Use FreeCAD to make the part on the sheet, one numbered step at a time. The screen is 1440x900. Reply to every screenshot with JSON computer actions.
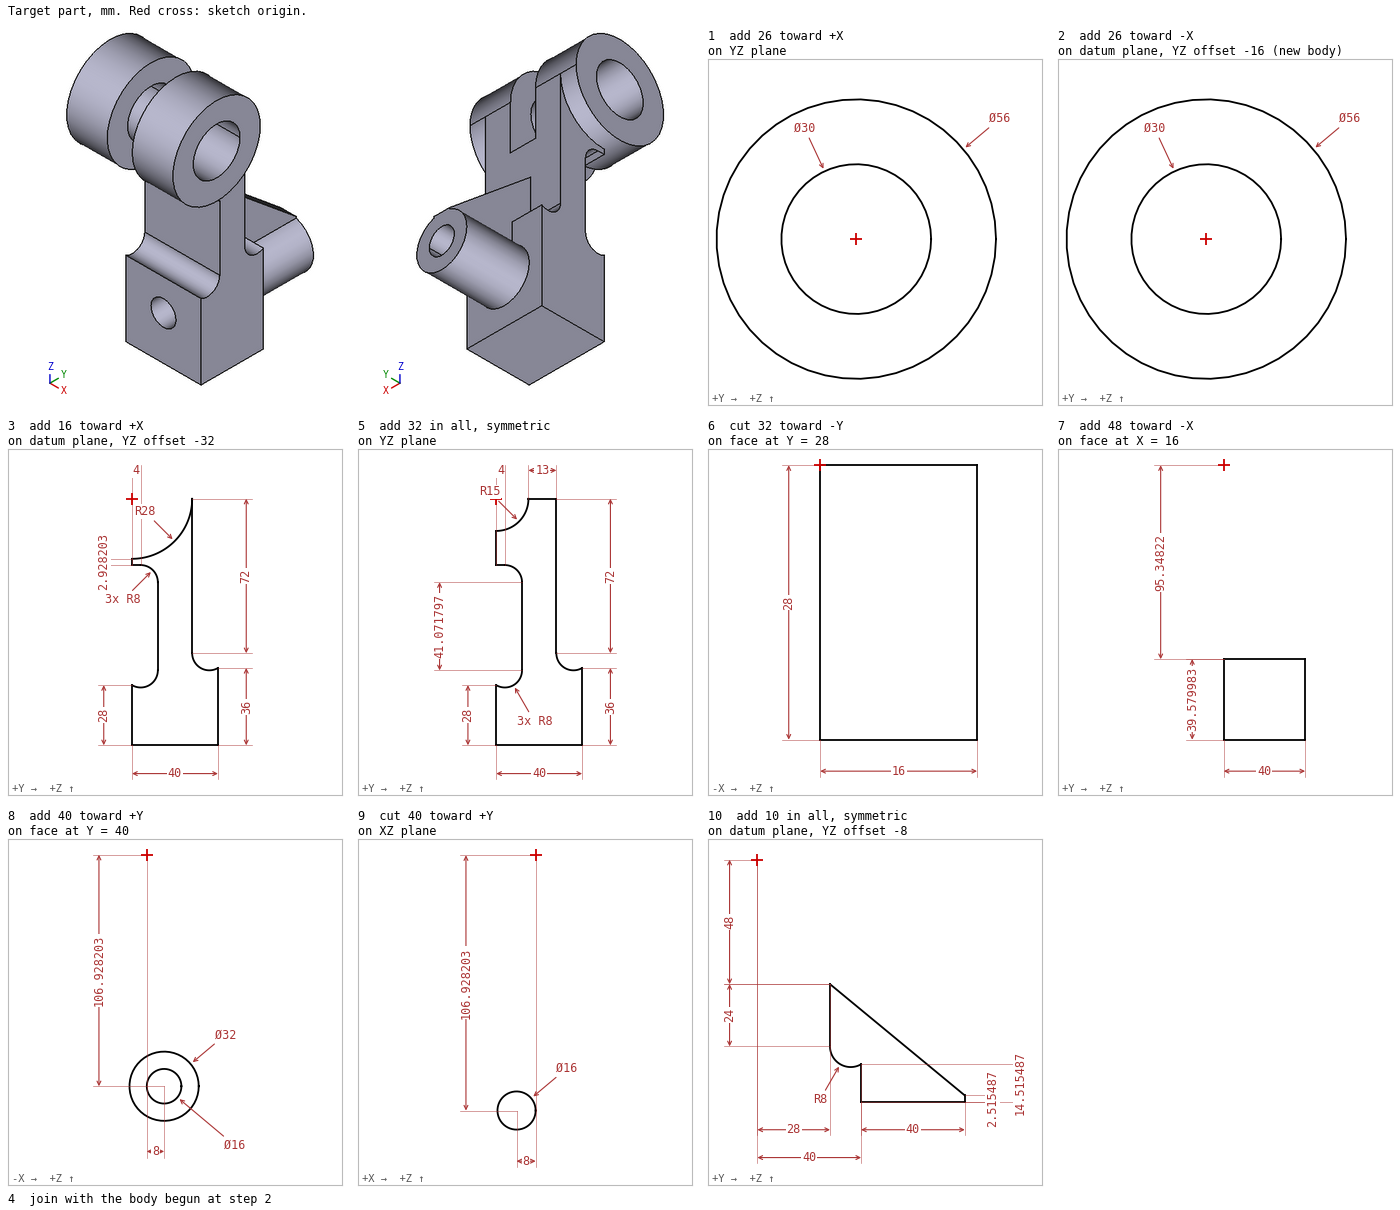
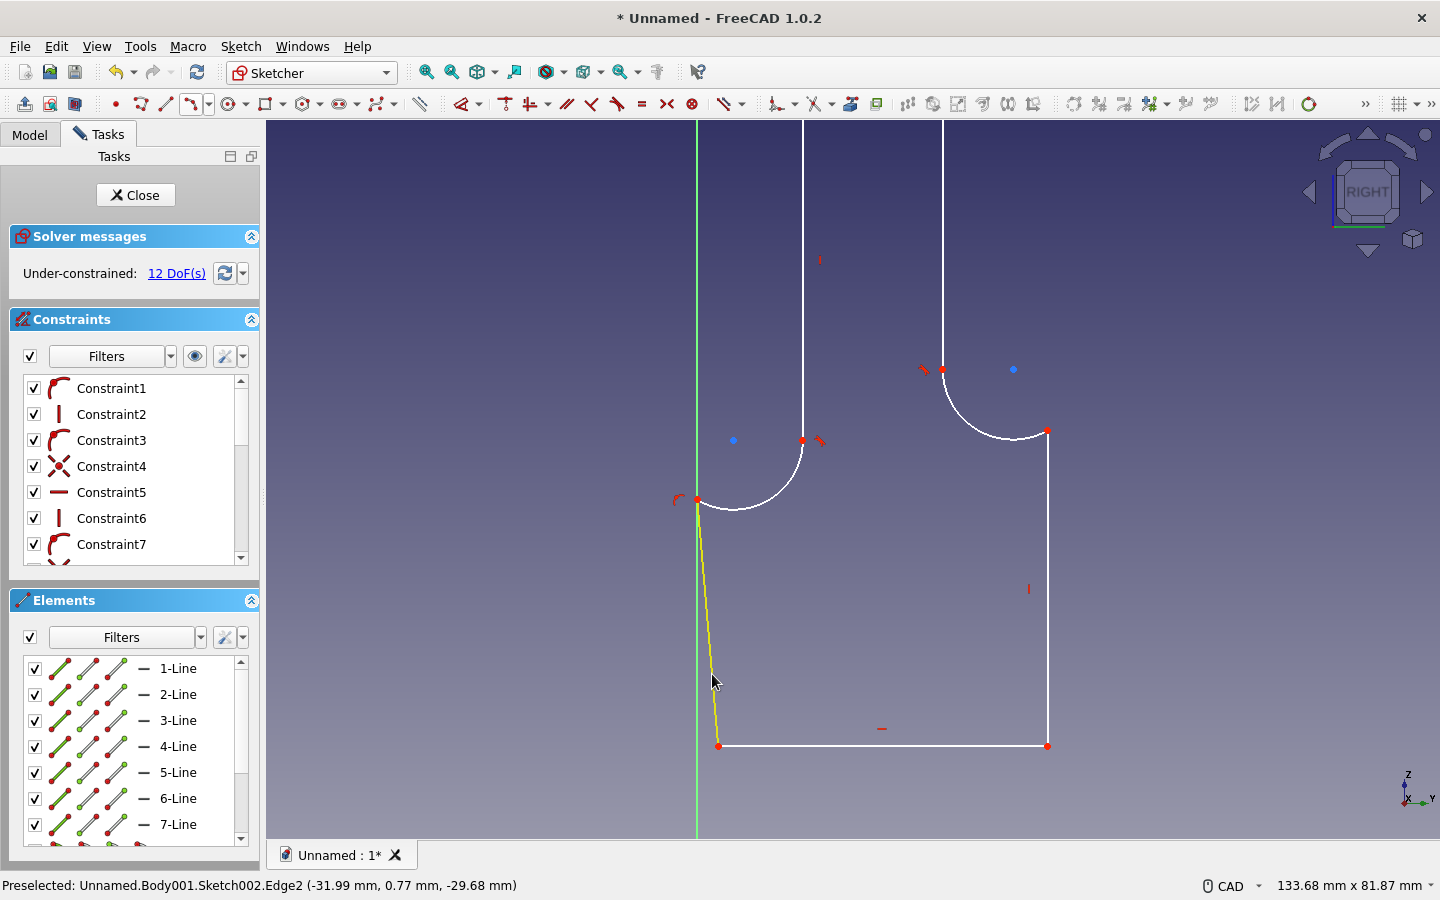
{"action": "left_click", "coordinate": [712, 672]}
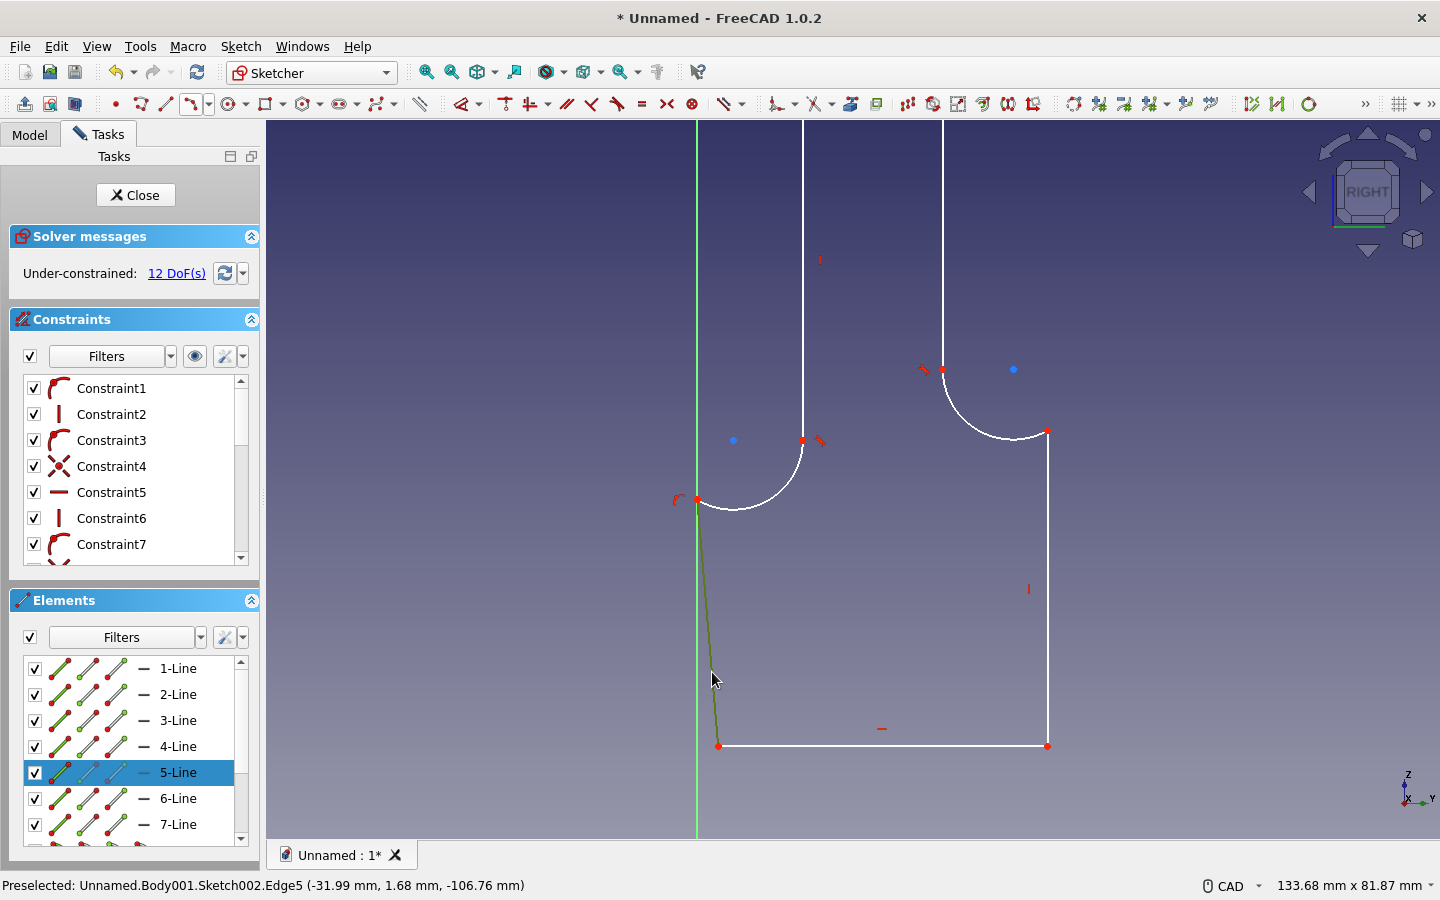
{"action": "left_click", "coordinate": [548, 104]}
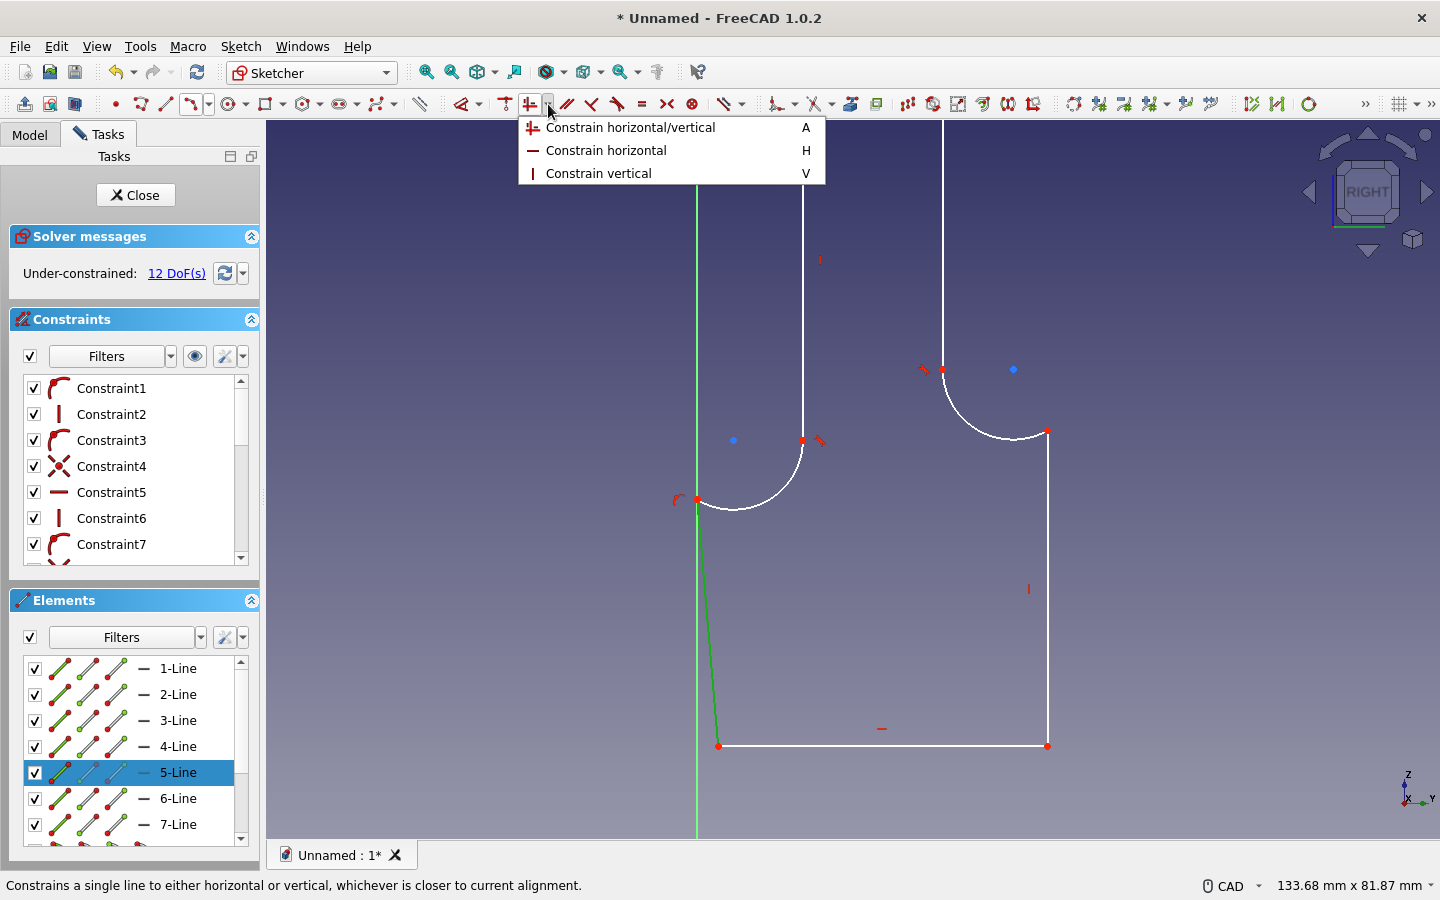
{"action": "left_click", "coordinate": [672, 174]}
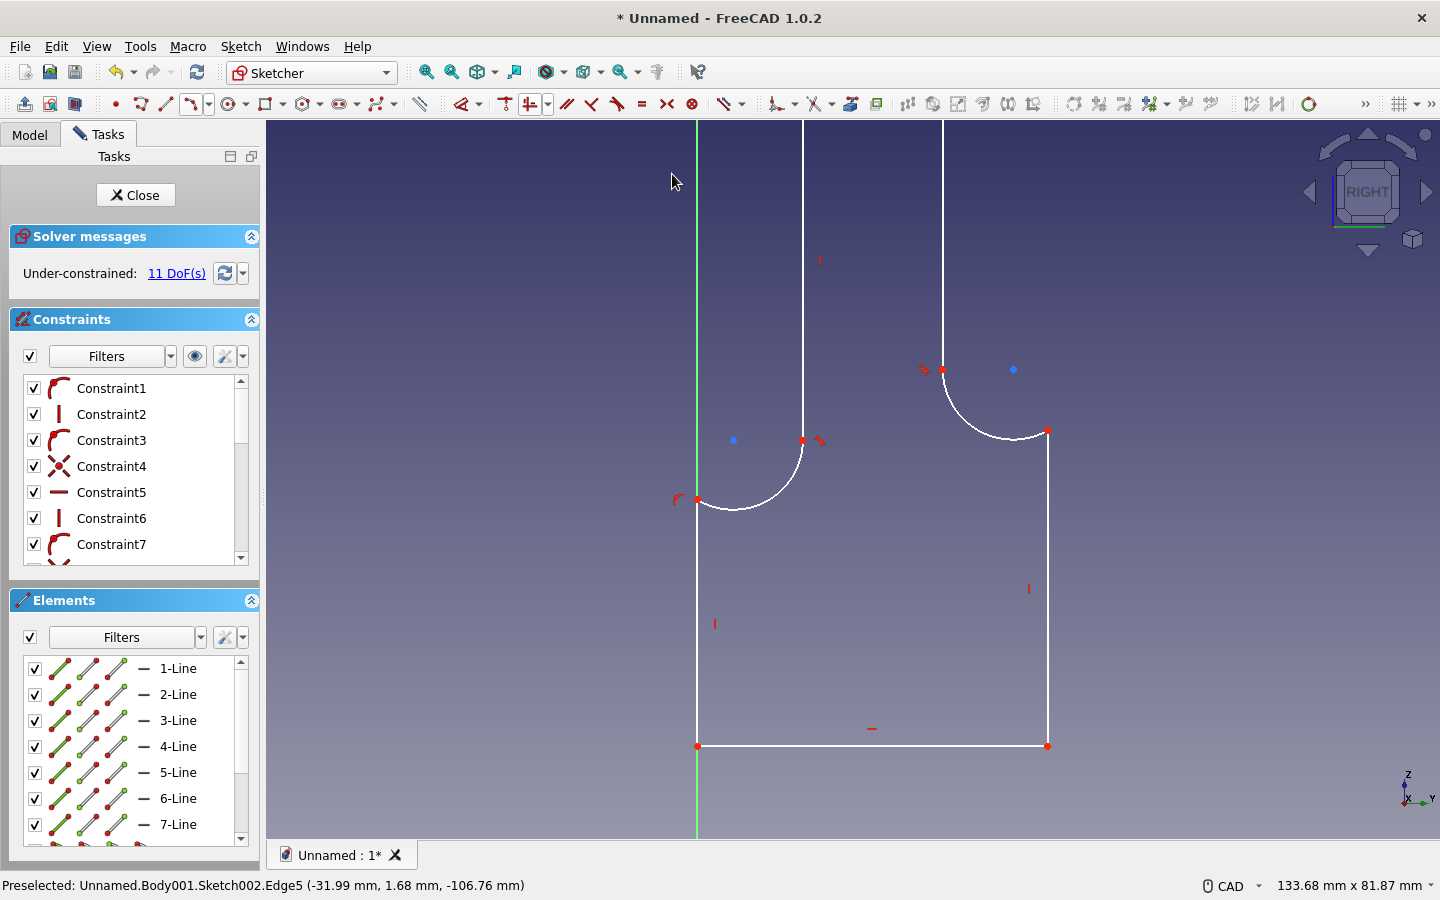
{"action": "scroll", "coordinate": [712, 675], "scroll_direction": "down", "scroll_amount": 4}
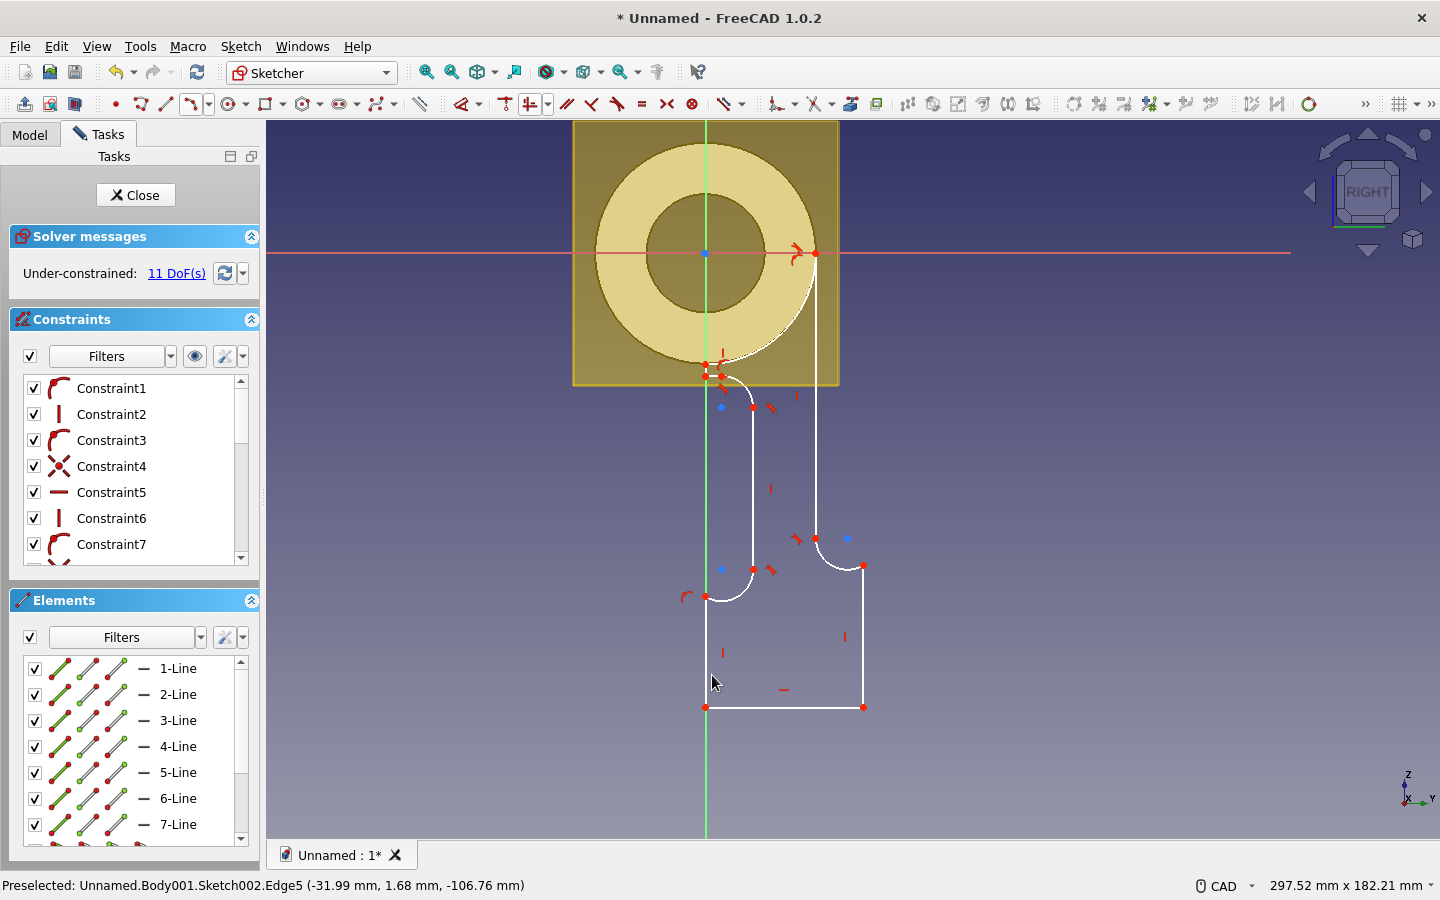
{"action": "left_click", "coordinate": [750, 393]}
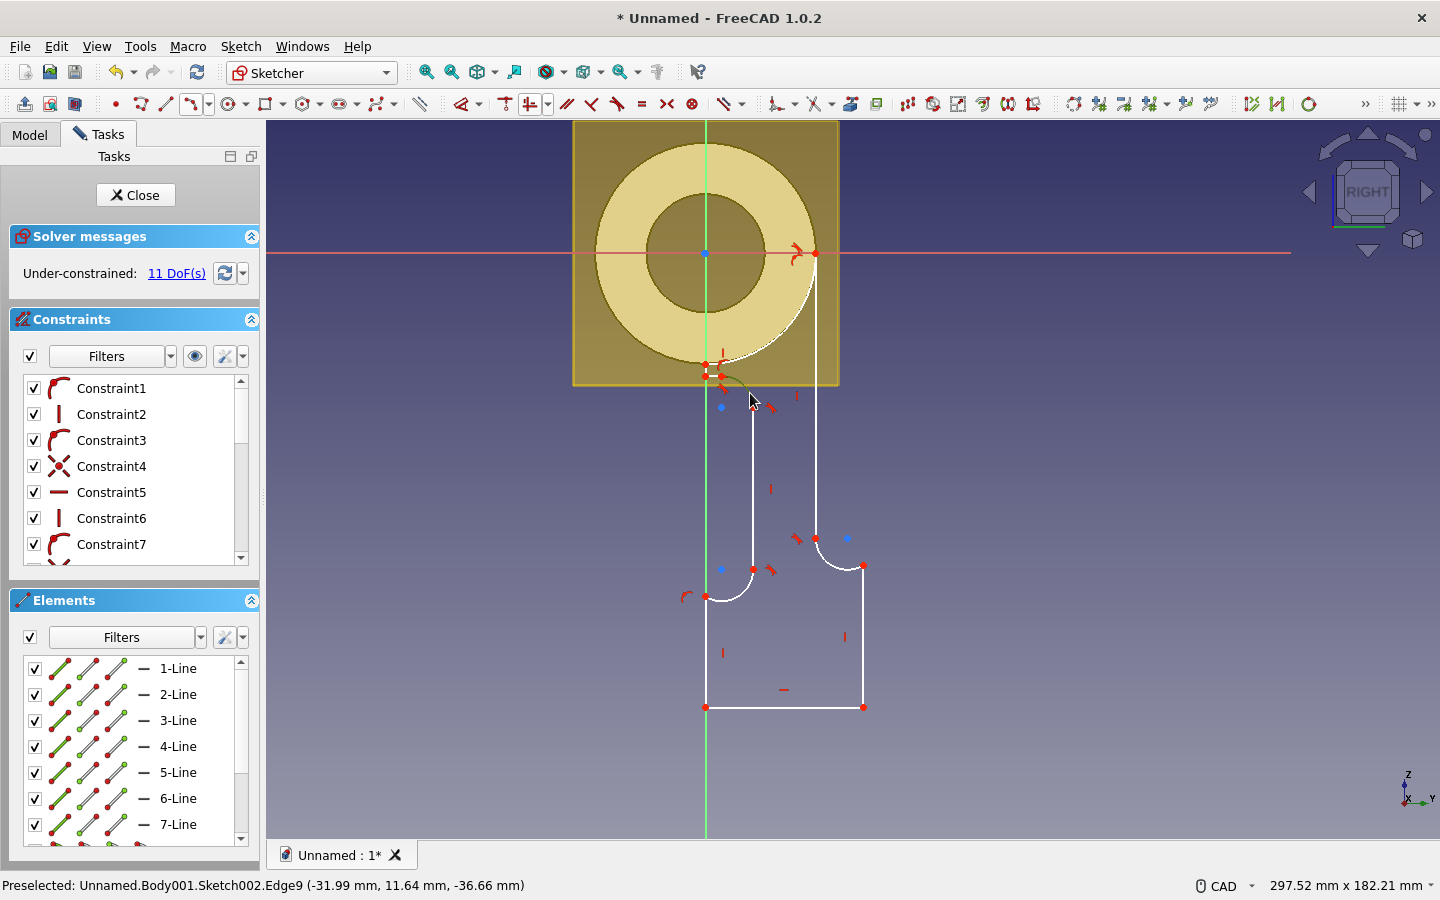
{"action": "left_click", "coordinate": [725, 601]}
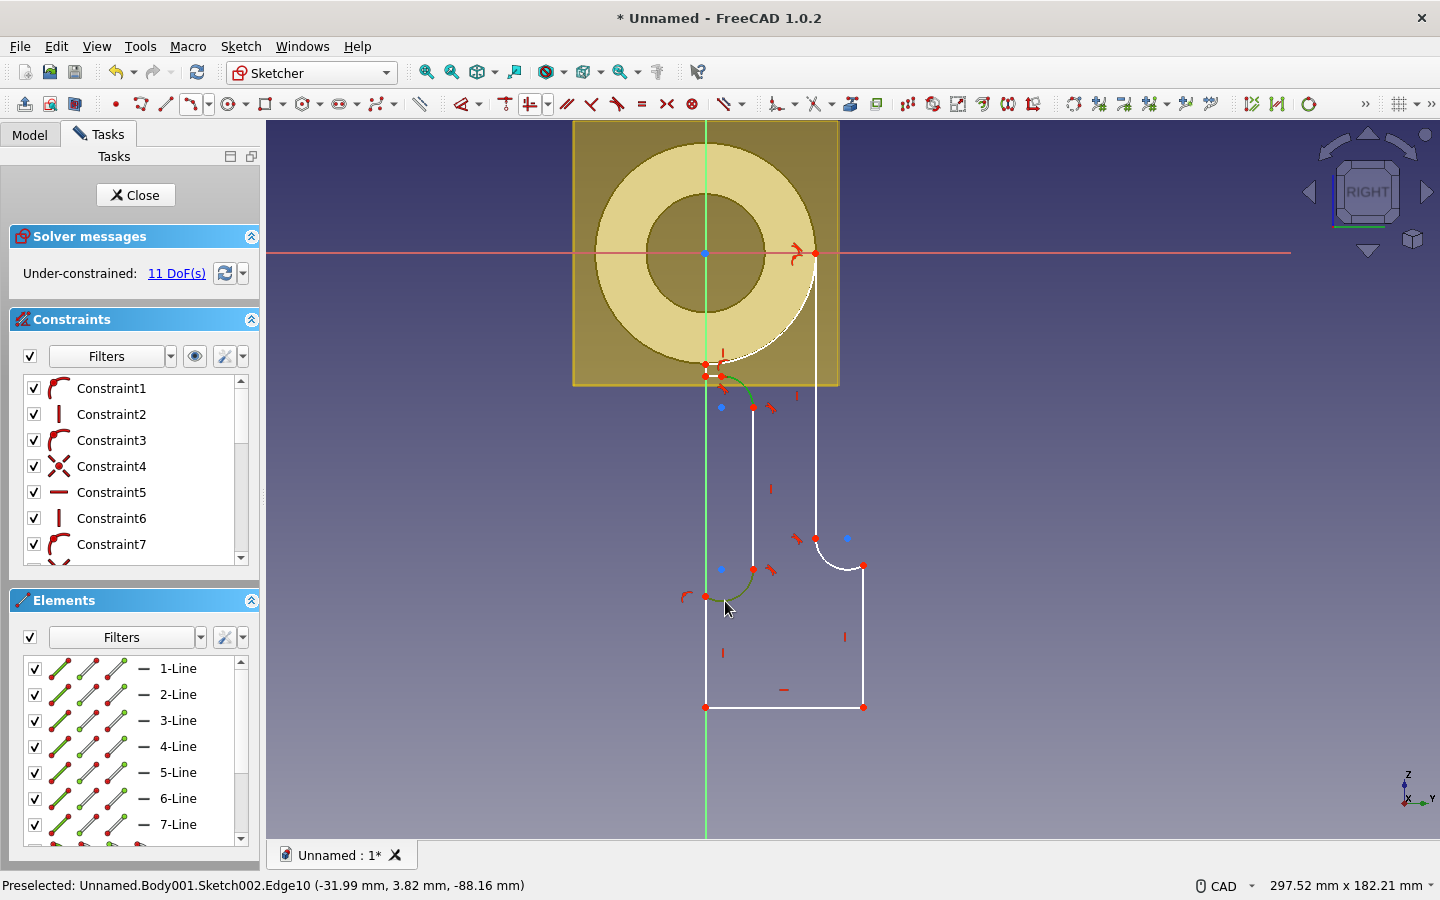
{"action": "left_click", "coordinate": [822, 557]}